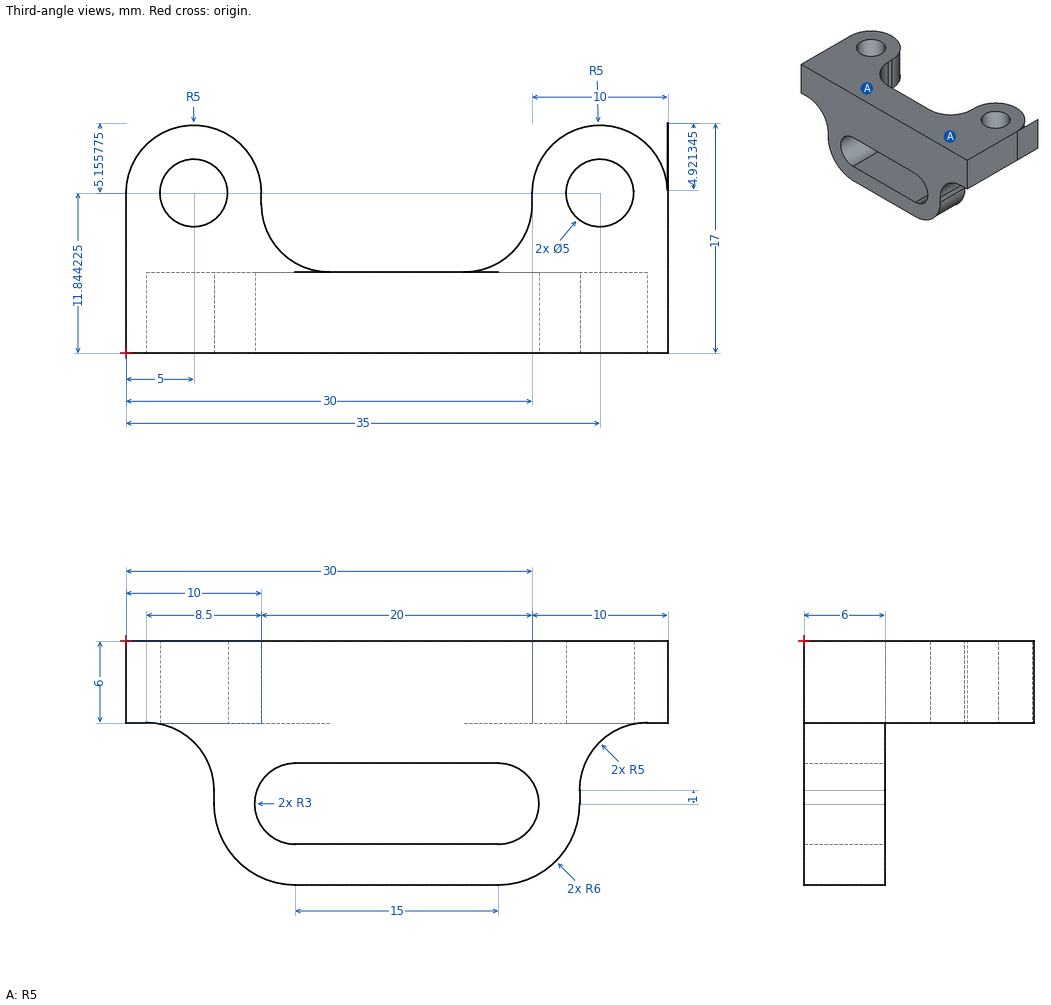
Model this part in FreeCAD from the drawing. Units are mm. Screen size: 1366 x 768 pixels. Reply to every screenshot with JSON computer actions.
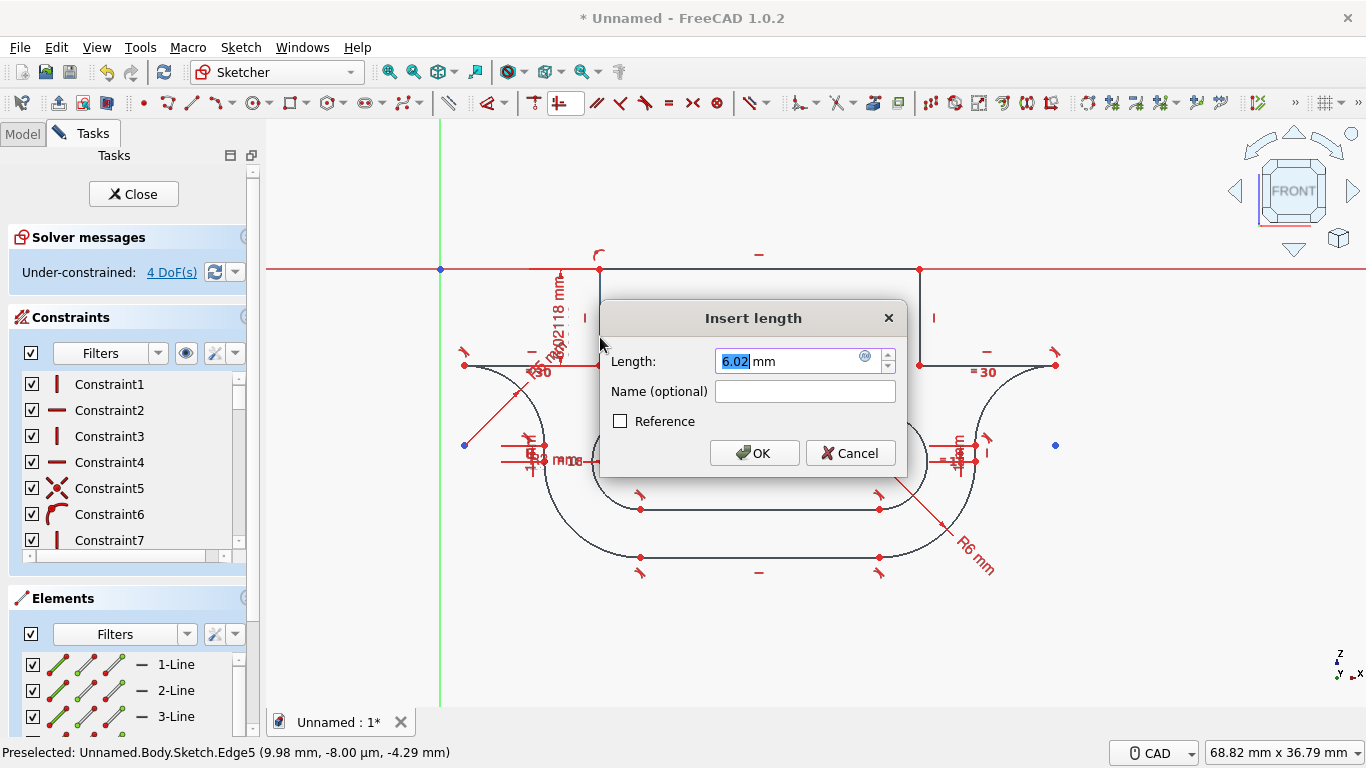
{"action": "type", "text": "6"}
{"action": "key", "text": "Return"}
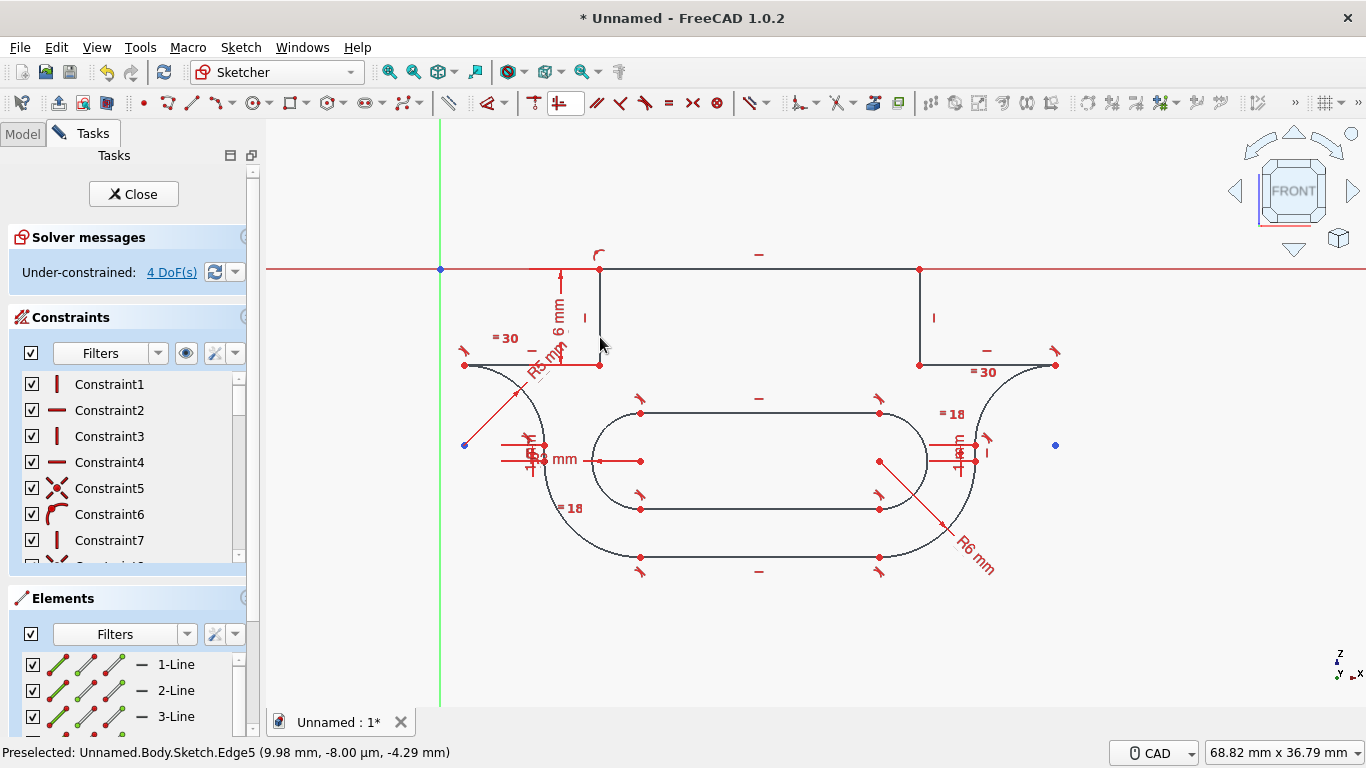
{"action": "left_click", "coordinate": [808, 557]}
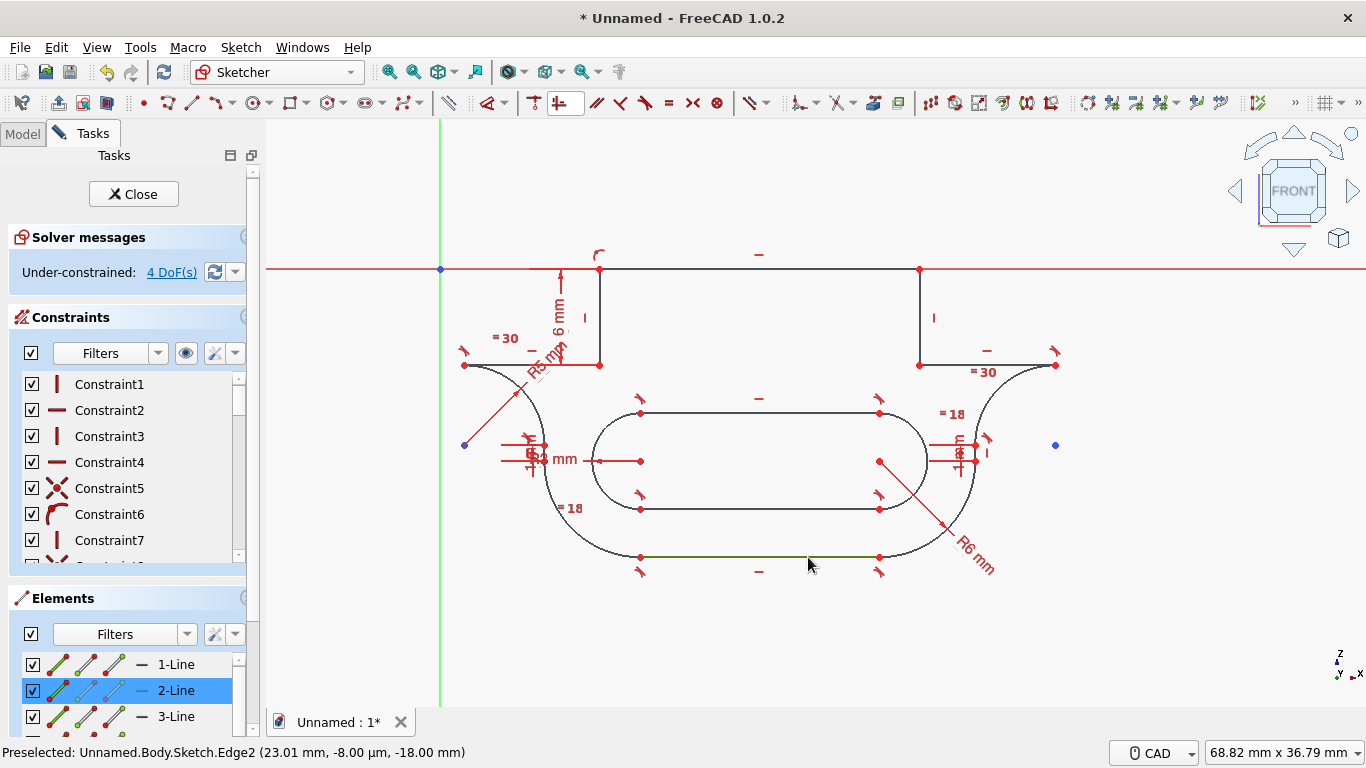
{"action": "key", "text": "l"}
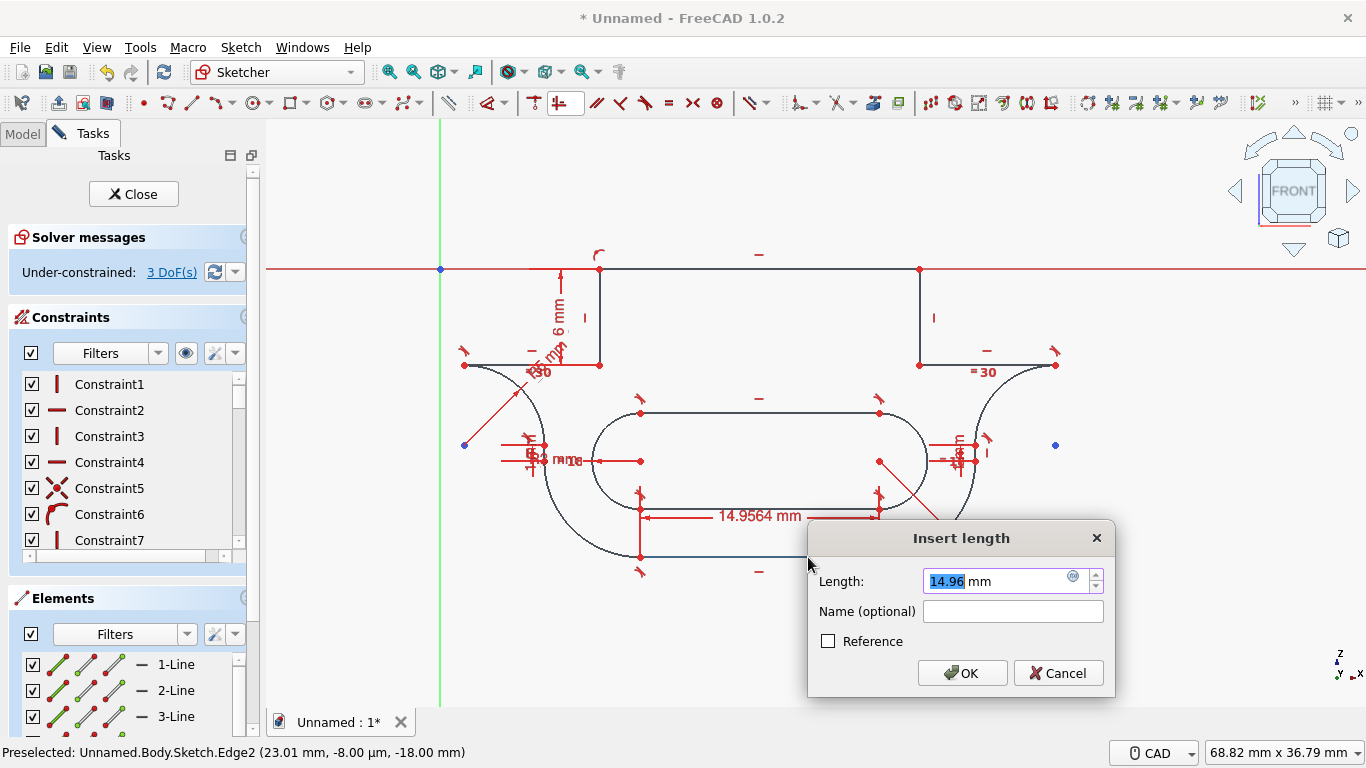
{"action": "type", "text": "15"}
{"action": "key", "text": "Return"}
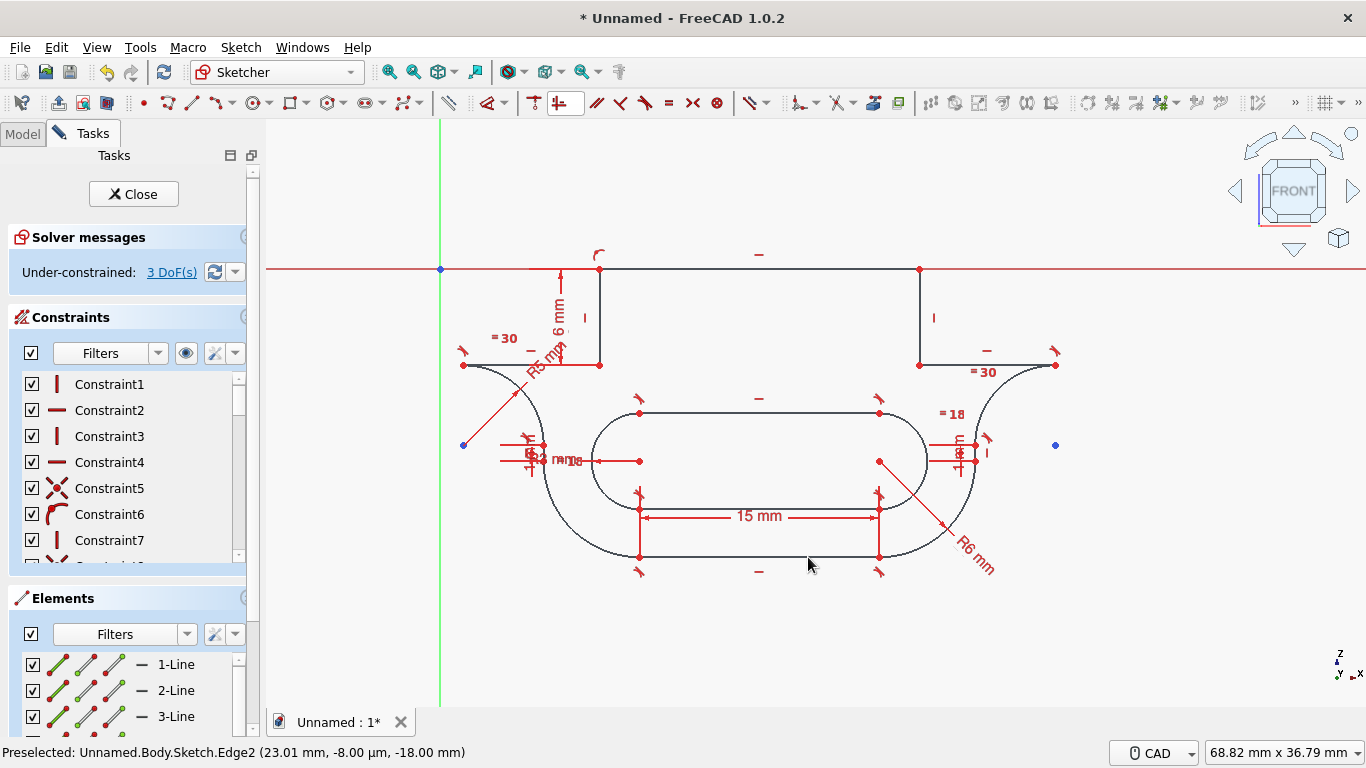
{"action": "left_click", "coordinate": [696, 269]}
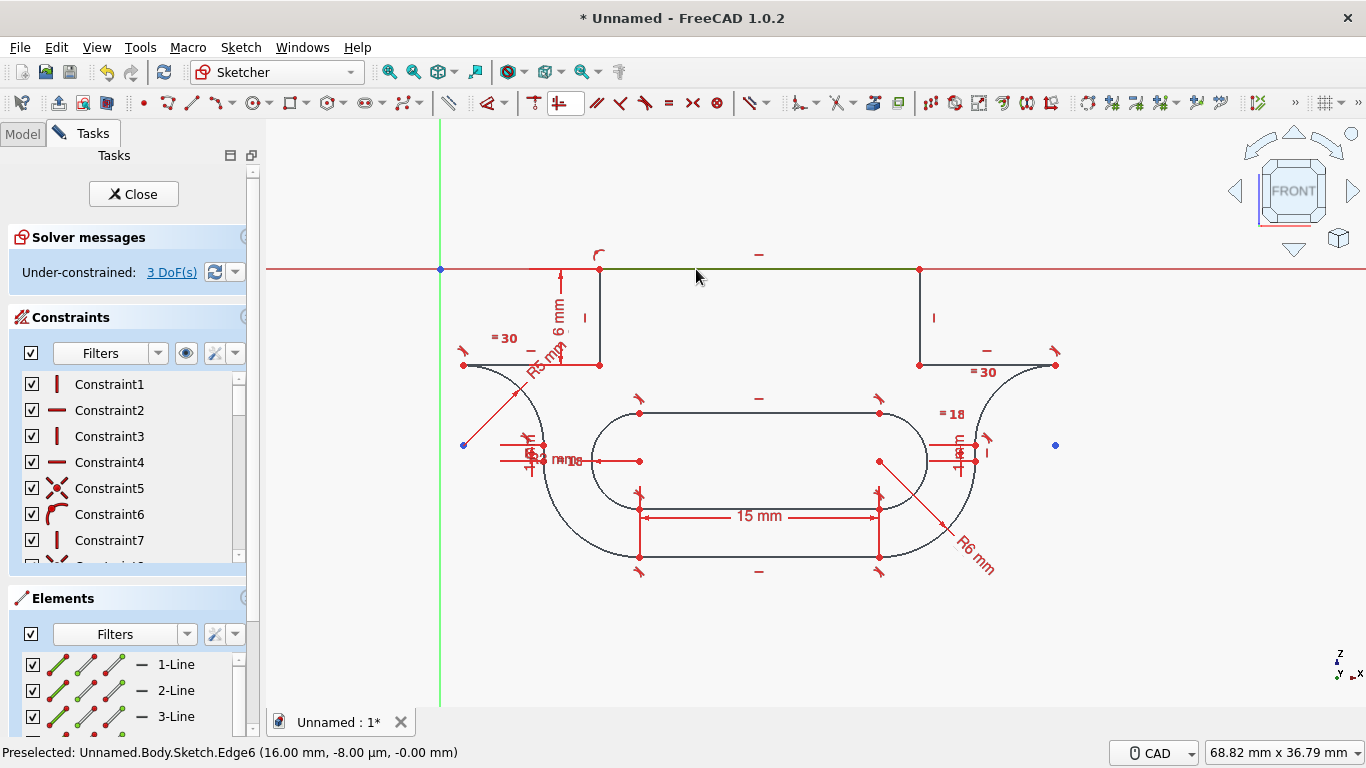
{"action": "key", "text": "l"}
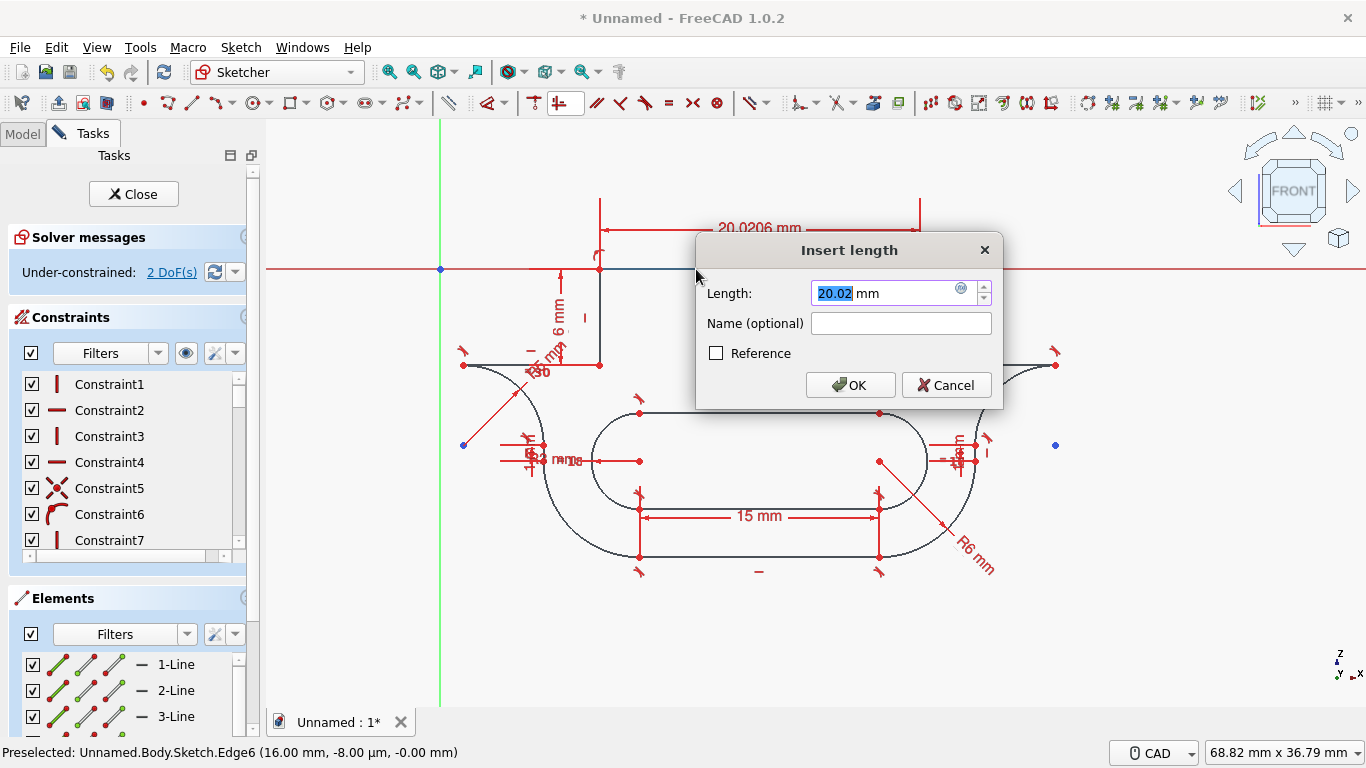
{"action": "type", "text": "20"}
{"action": "key", "text": "Return"}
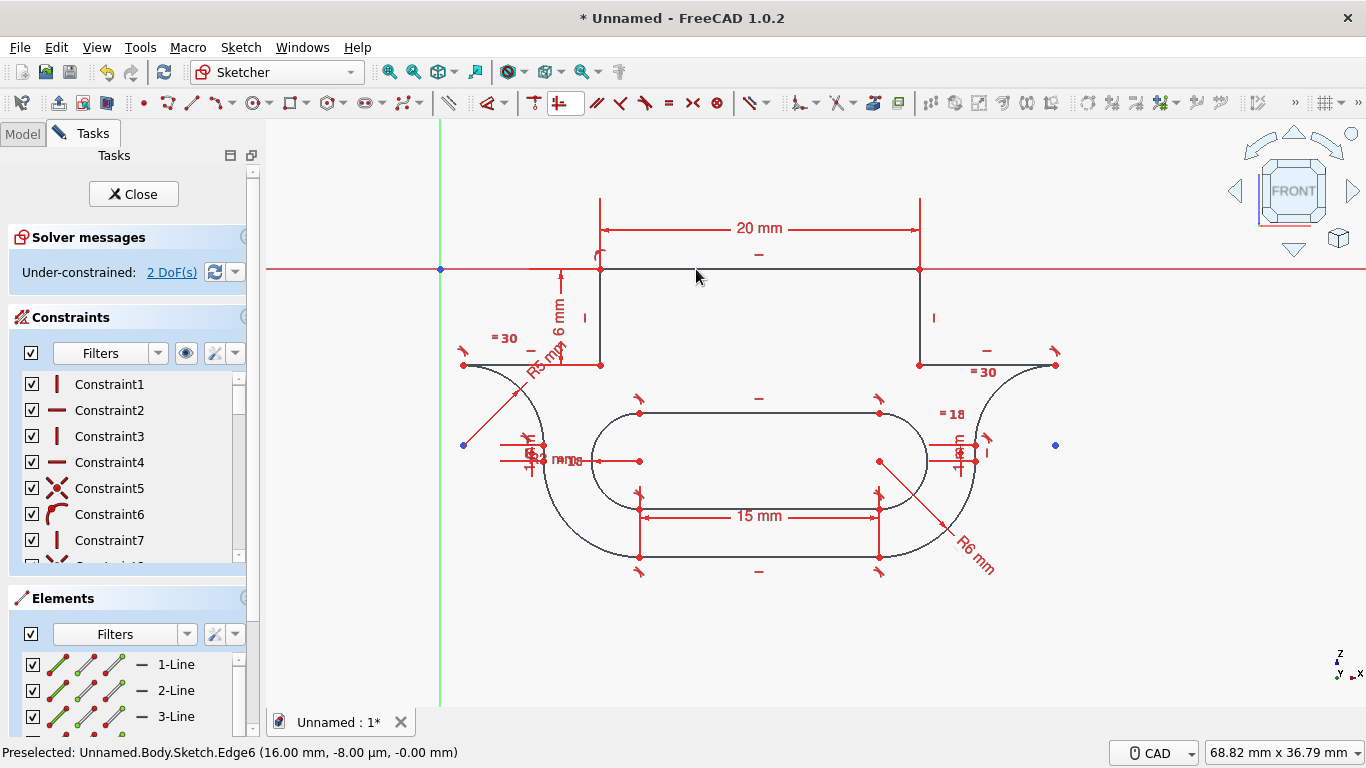
{"action": "scroll", "coordinate": [505, 365], "scroll_direction": "up", "scroll_amount": 2}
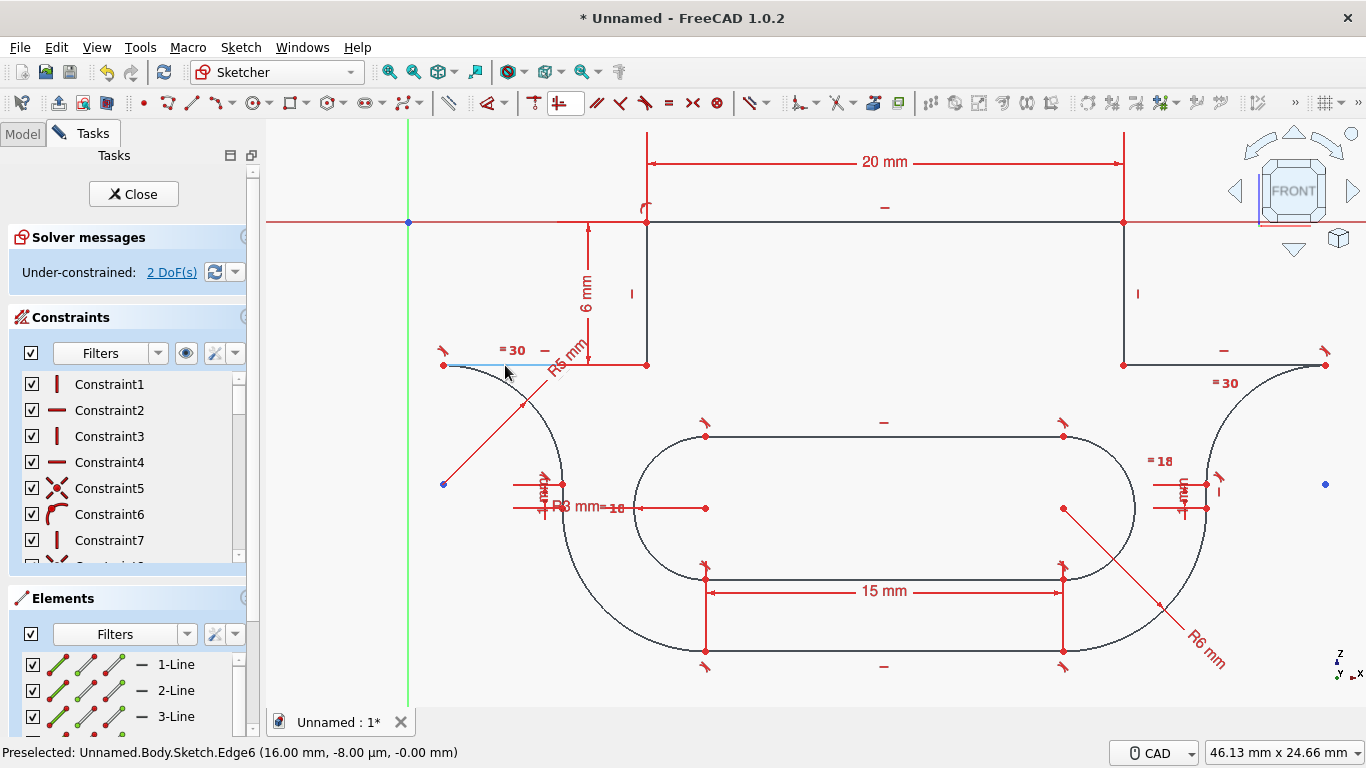
{"action": "left_click", "coordinate": [504, 365]}